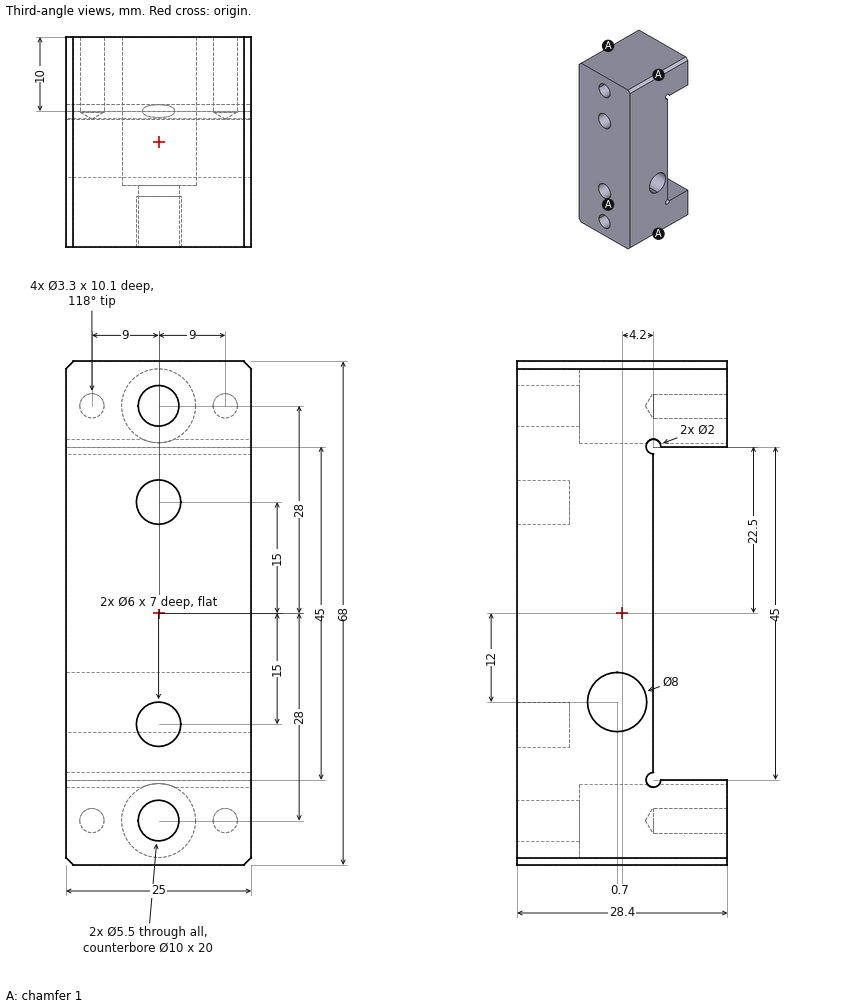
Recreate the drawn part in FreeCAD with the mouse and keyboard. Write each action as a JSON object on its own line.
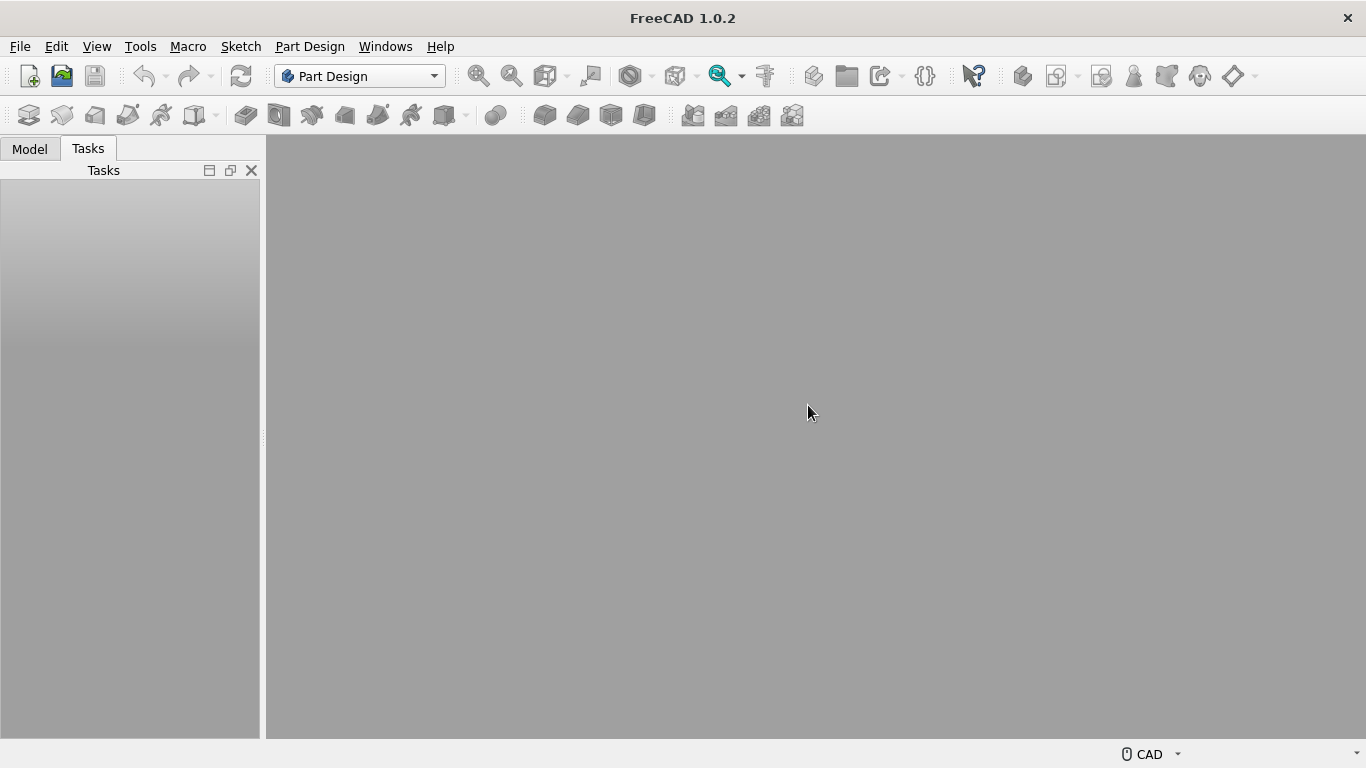
{"action": "key", "text": "ctrl+n"}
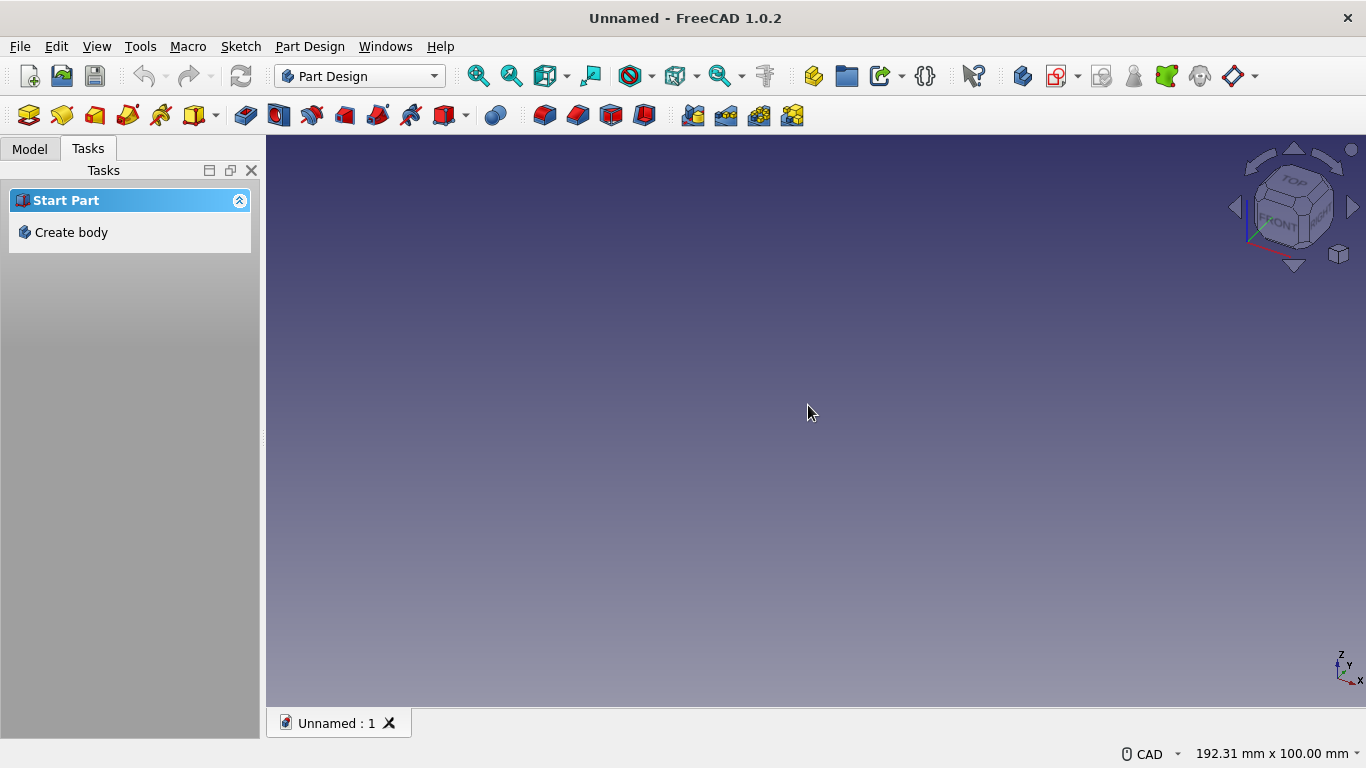
{"action": "left_click", "coordinate": [1056, 76]}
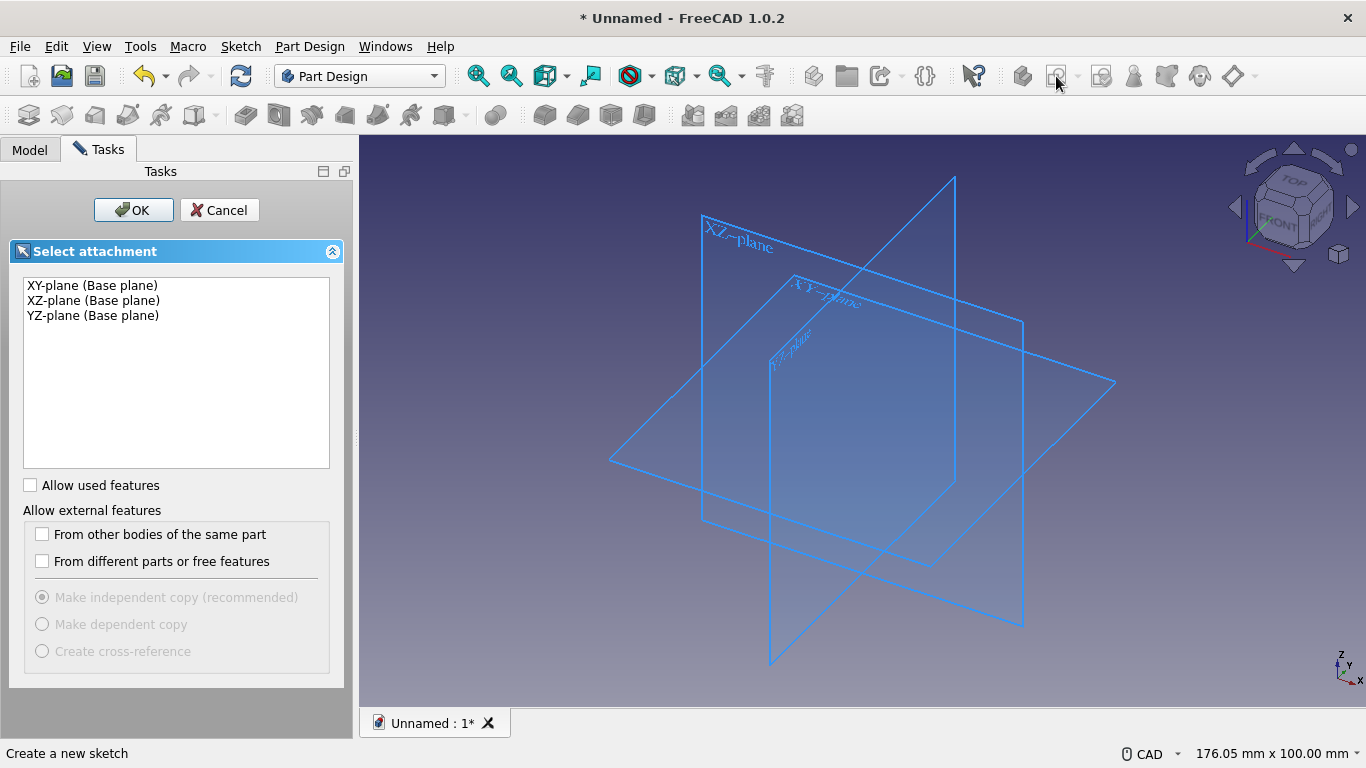
{"action": "left_click", "coordinate": [84, 300]}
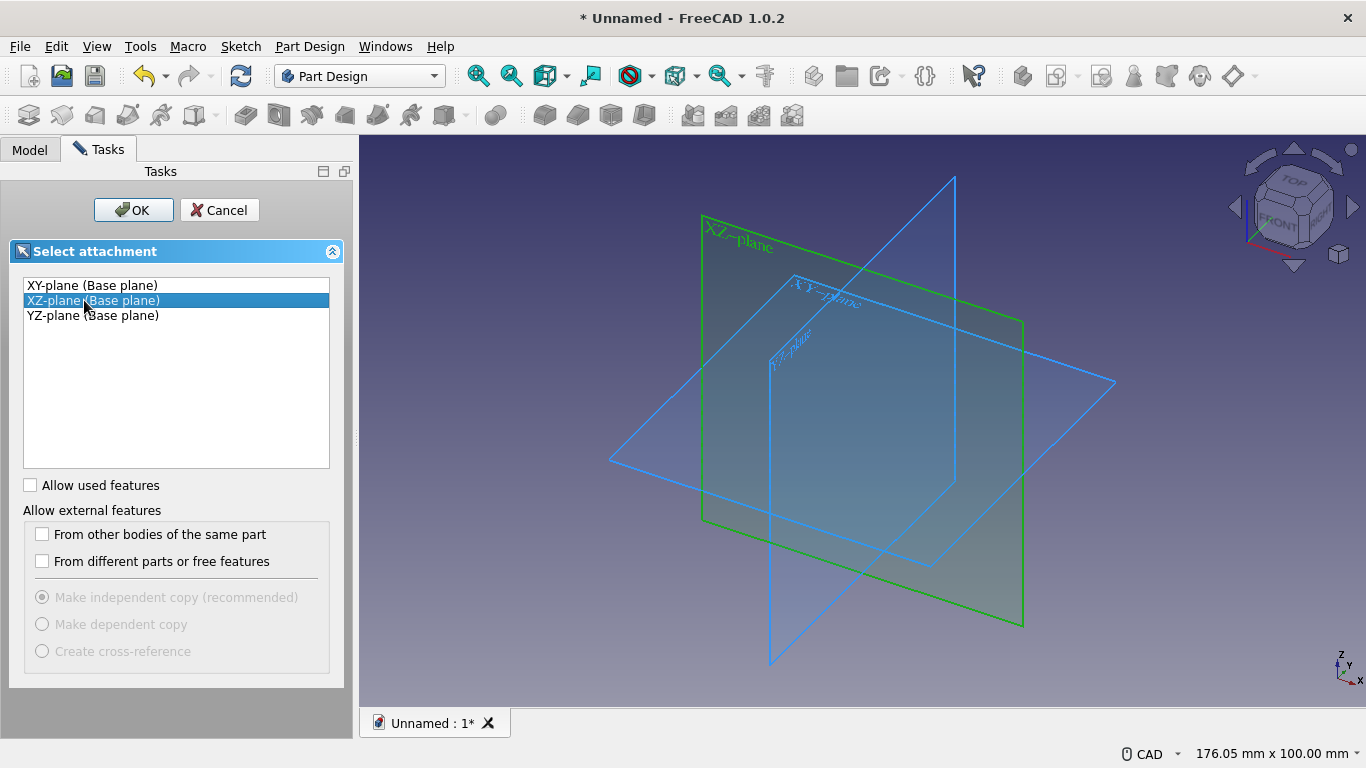
{"action": "left_click", "coordinate": [134, 210]}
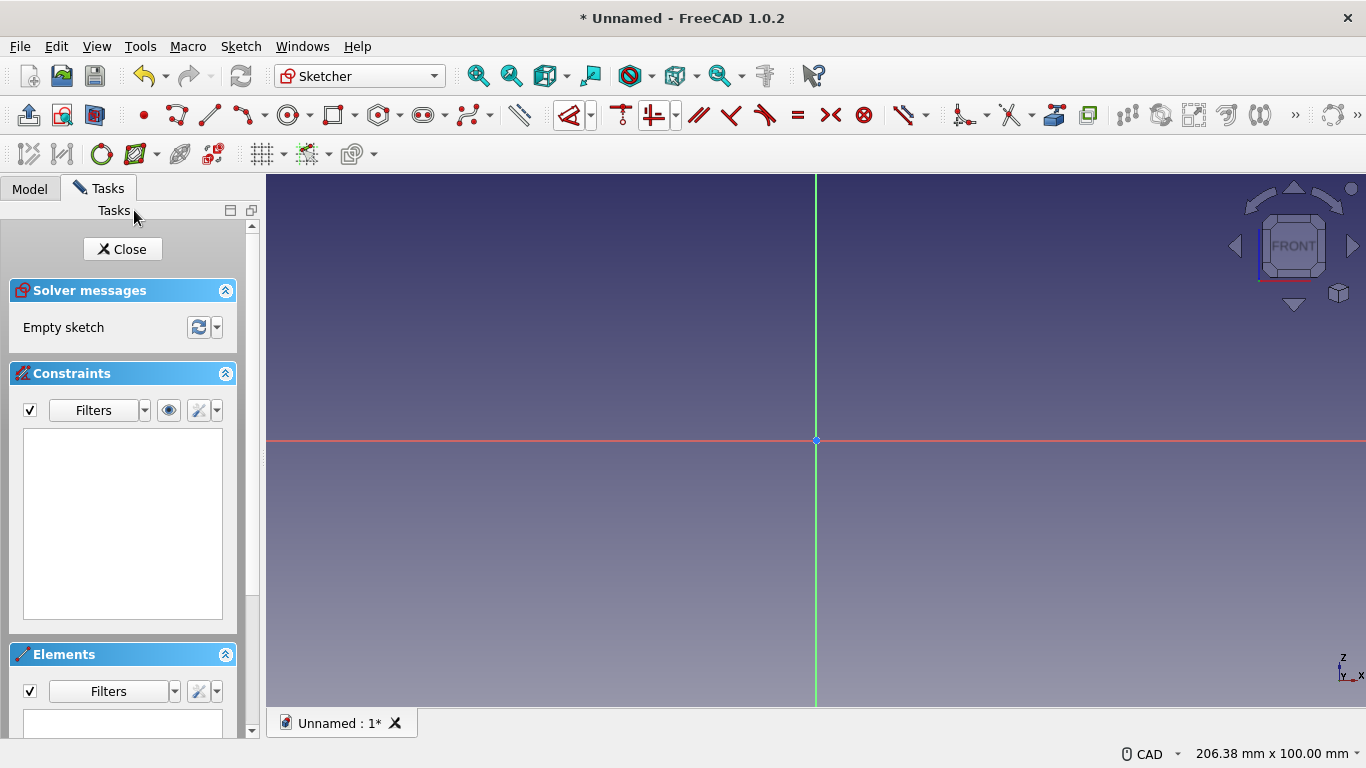
{"action": "key", "text": "g v"}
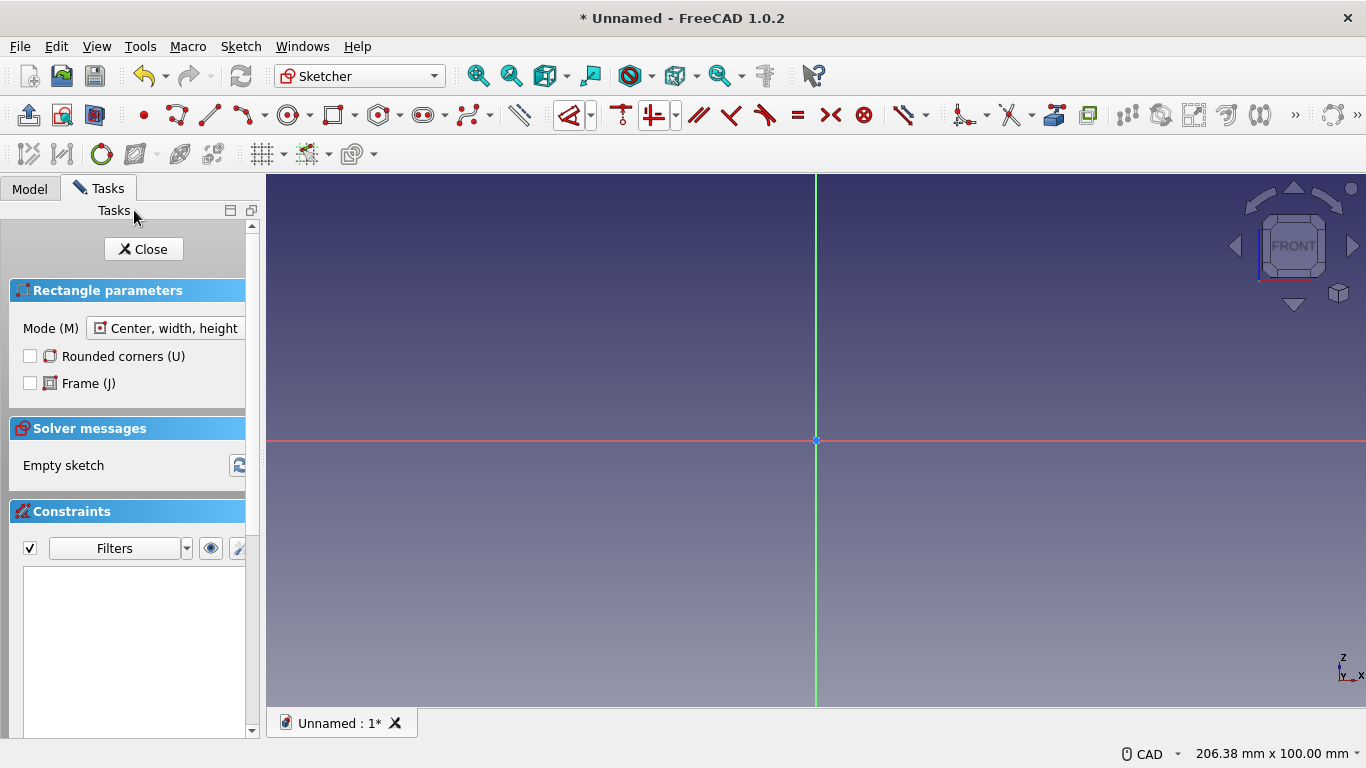
{"action": "left_click", "coordinate": [816, 440]}
{"action": "left_click", "coordinate": [883, 259]}
{"action": "key", "text": "Escape"}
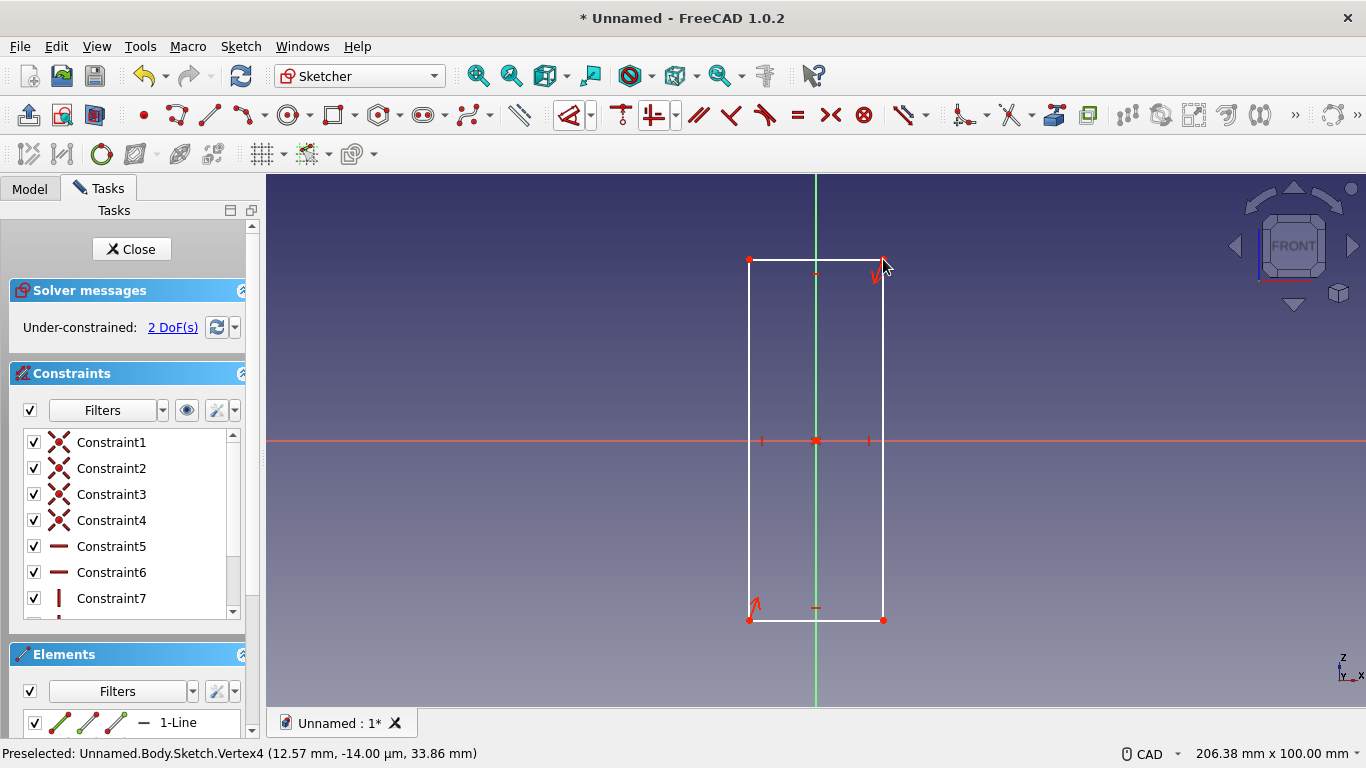
{"action": "key", "text": "d"}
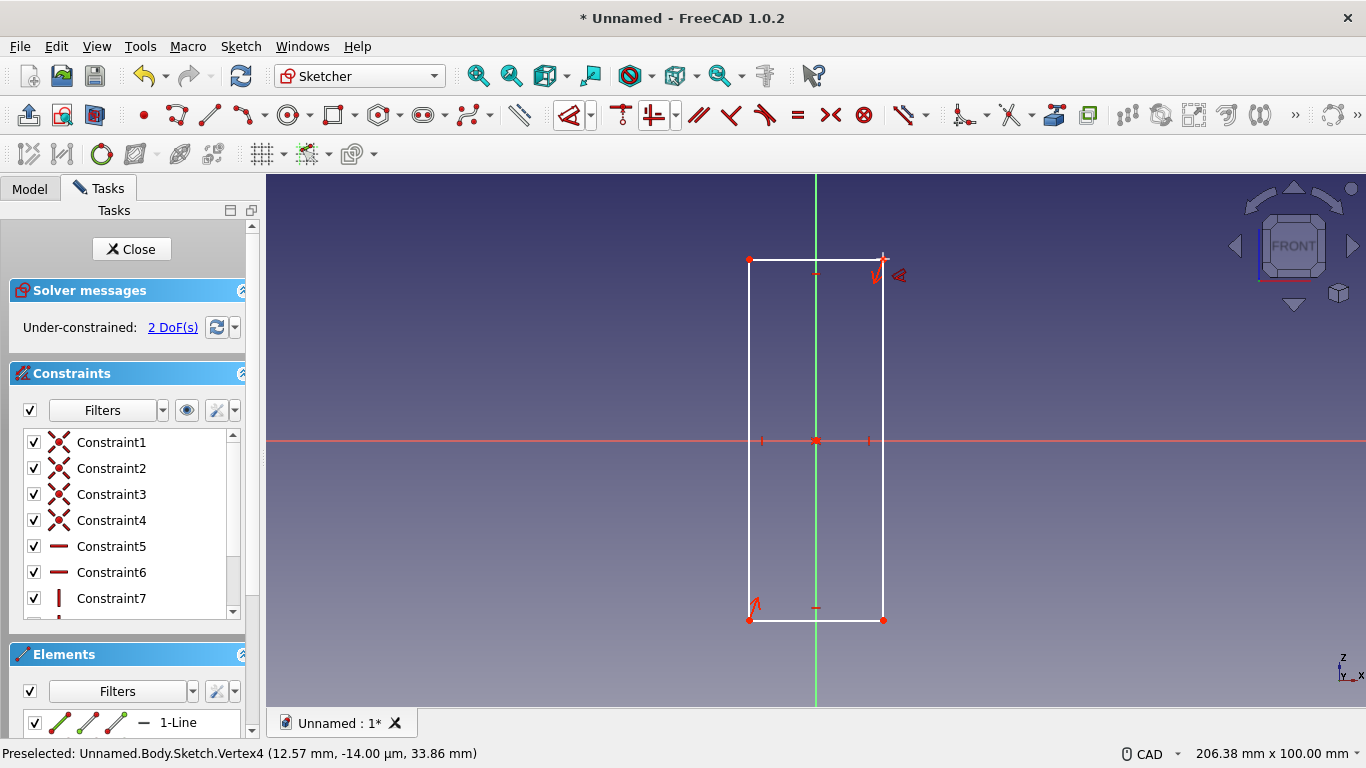
{"action": "left_click", "coordinate": [789, 621]}
{"action": "left_click", "coordinate": [785, 655]}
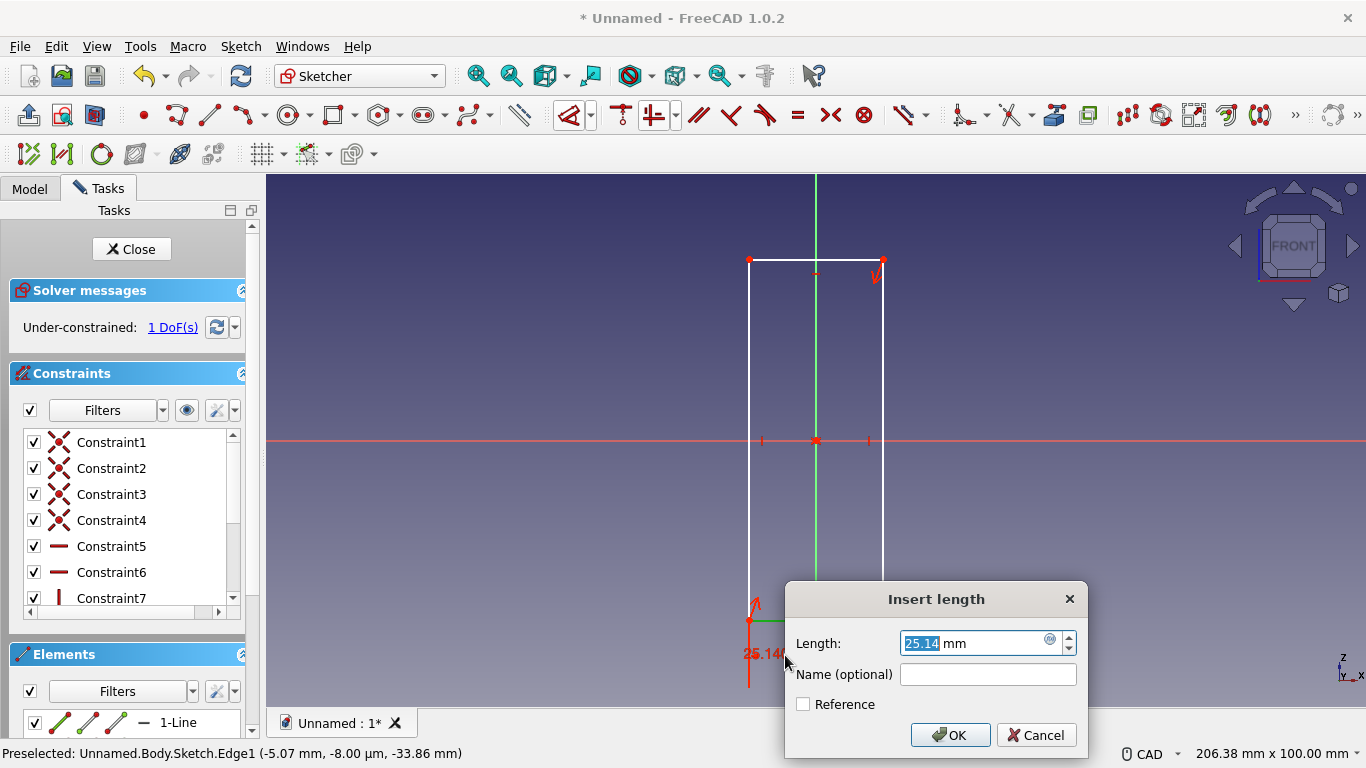
{"action": "type", "text": "25"}
{"action": "key", "text": "Return"}